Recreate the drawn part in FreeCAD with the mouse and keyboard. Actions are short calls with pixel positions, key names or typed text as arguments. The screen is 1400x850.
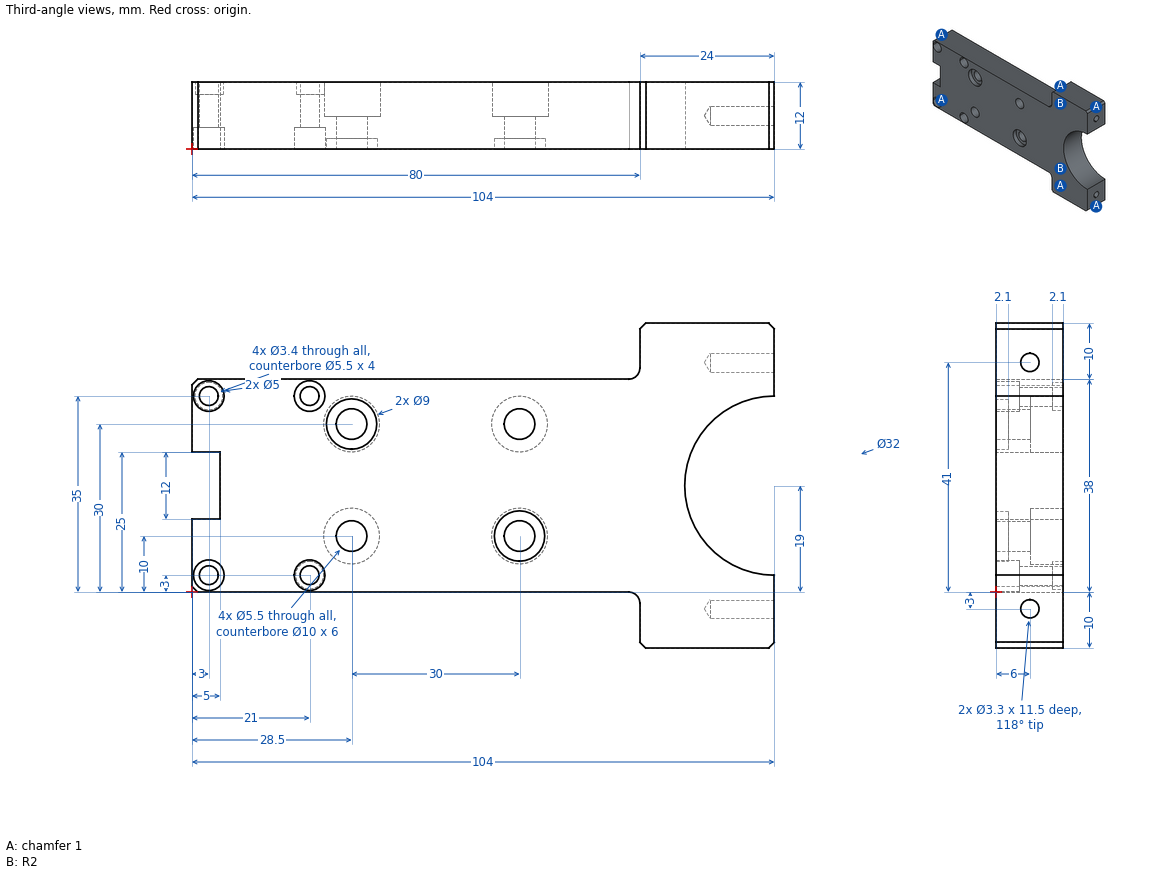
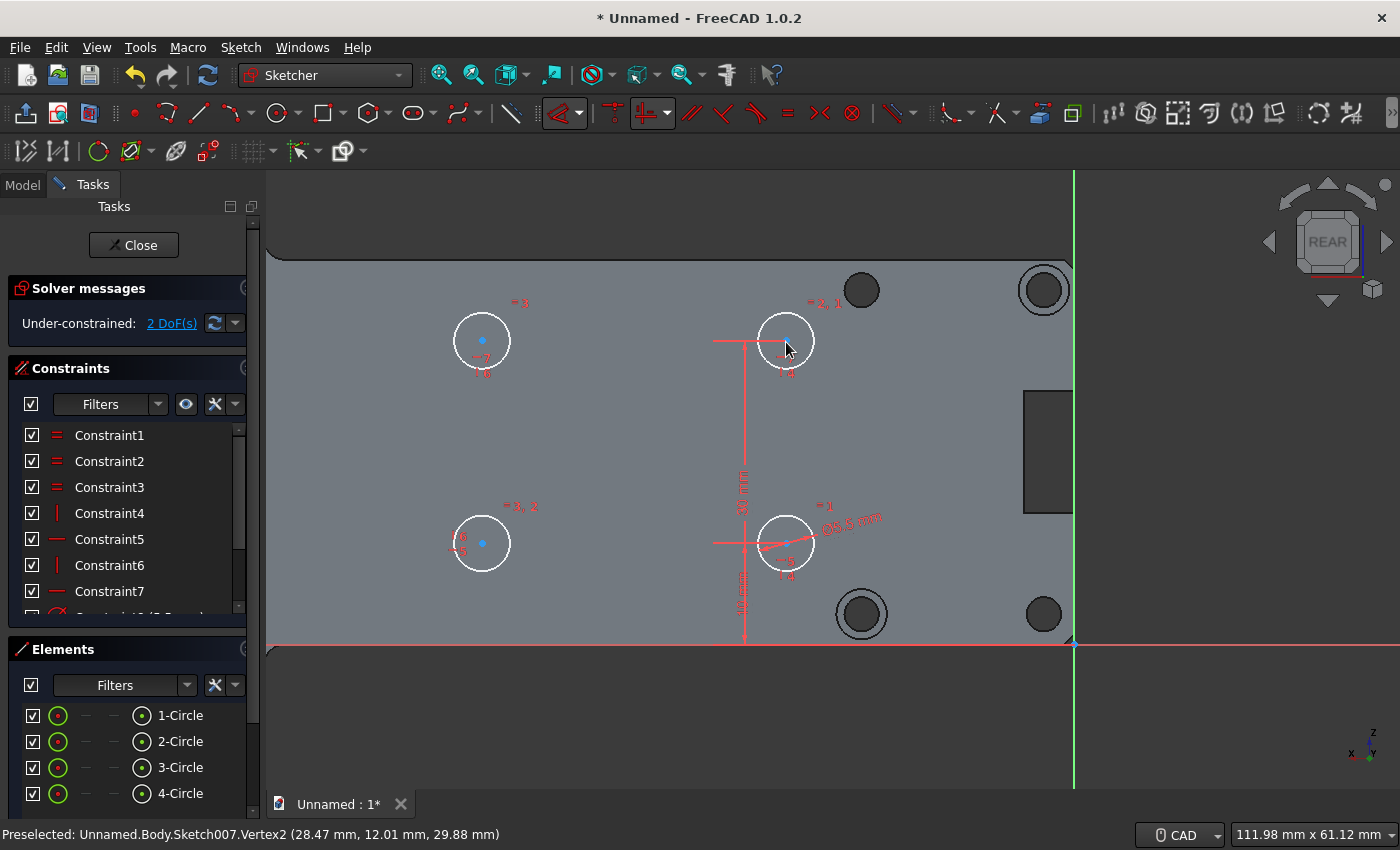
click(786, 543)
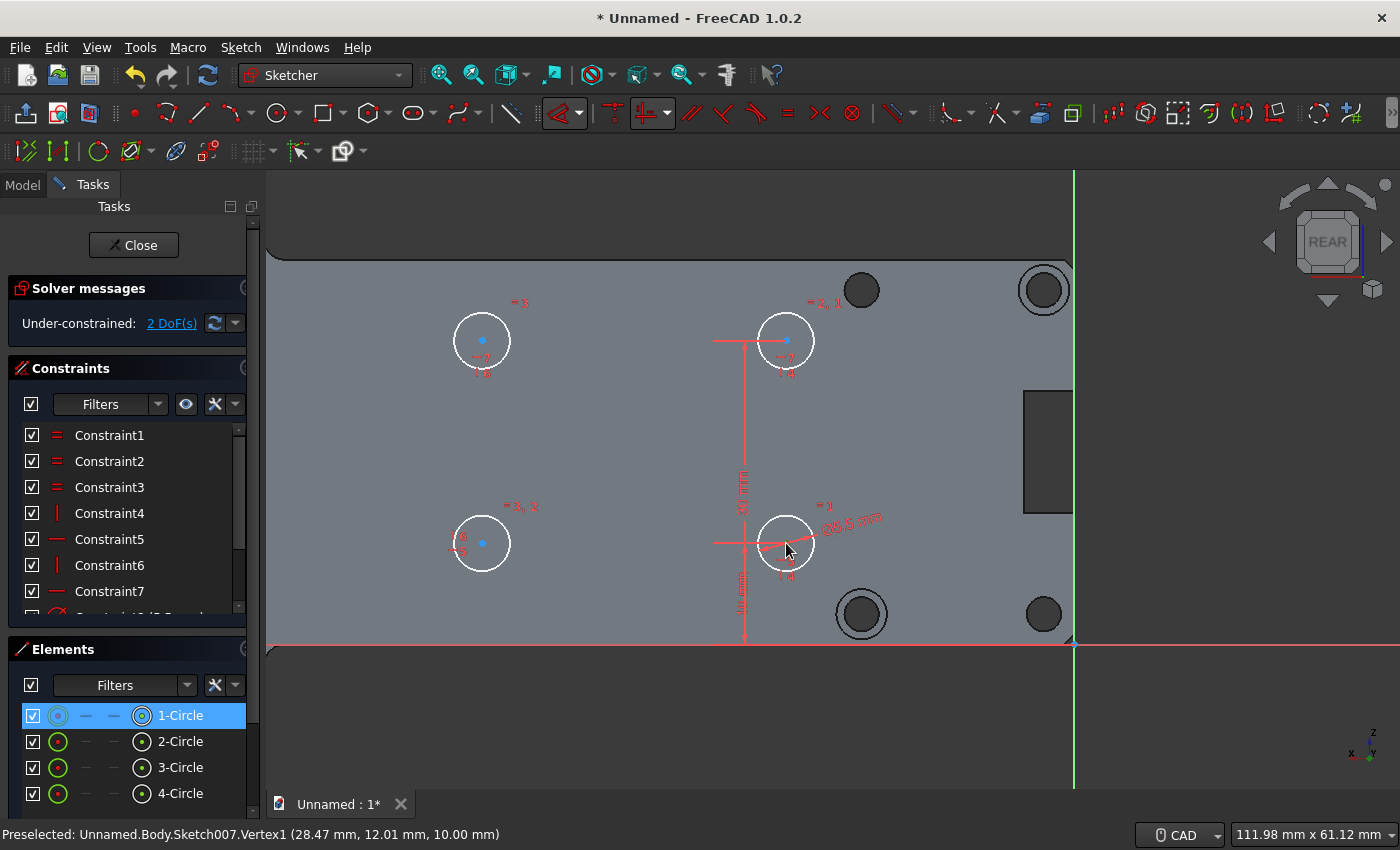
click(482, 543)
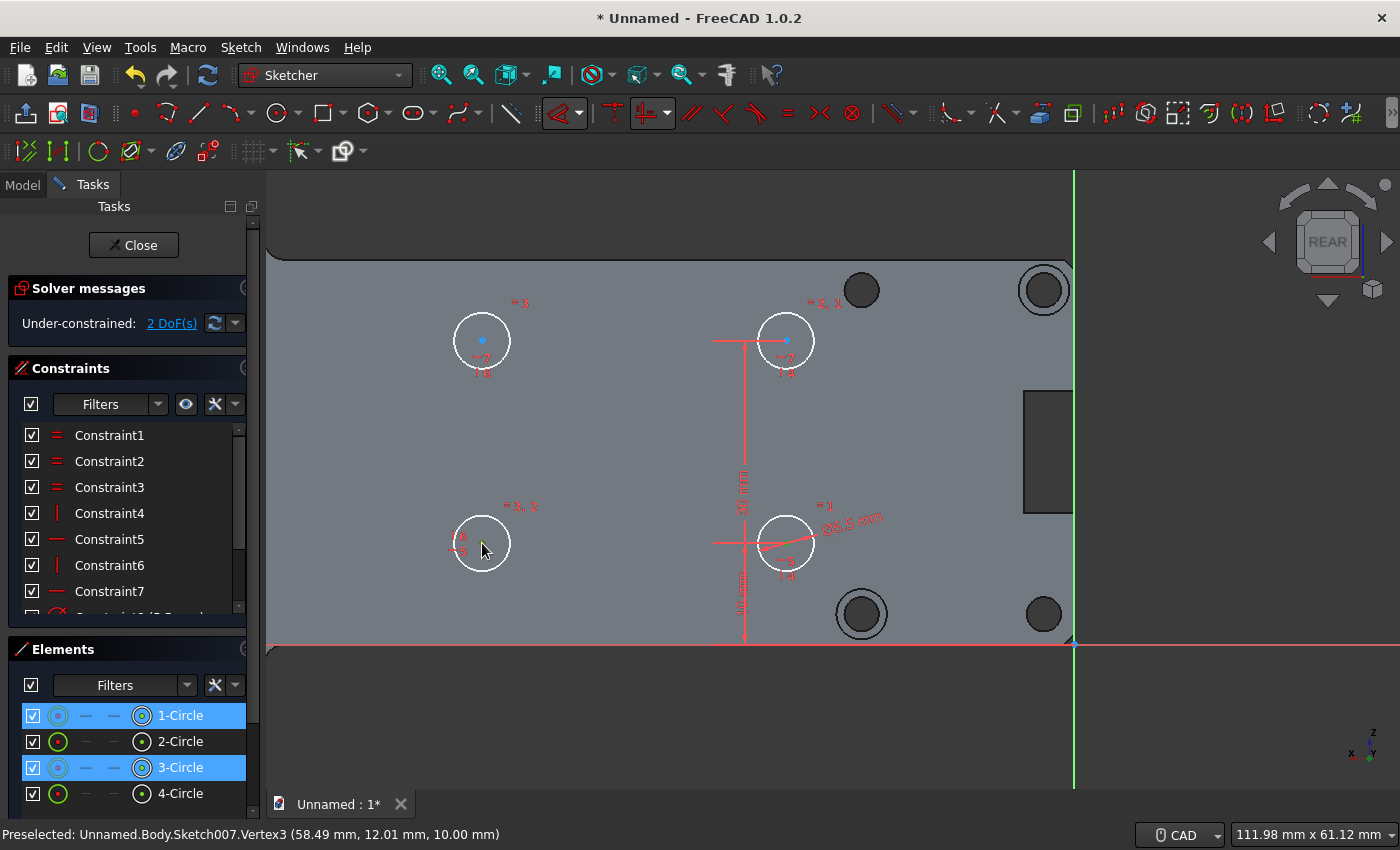
click(582, 114)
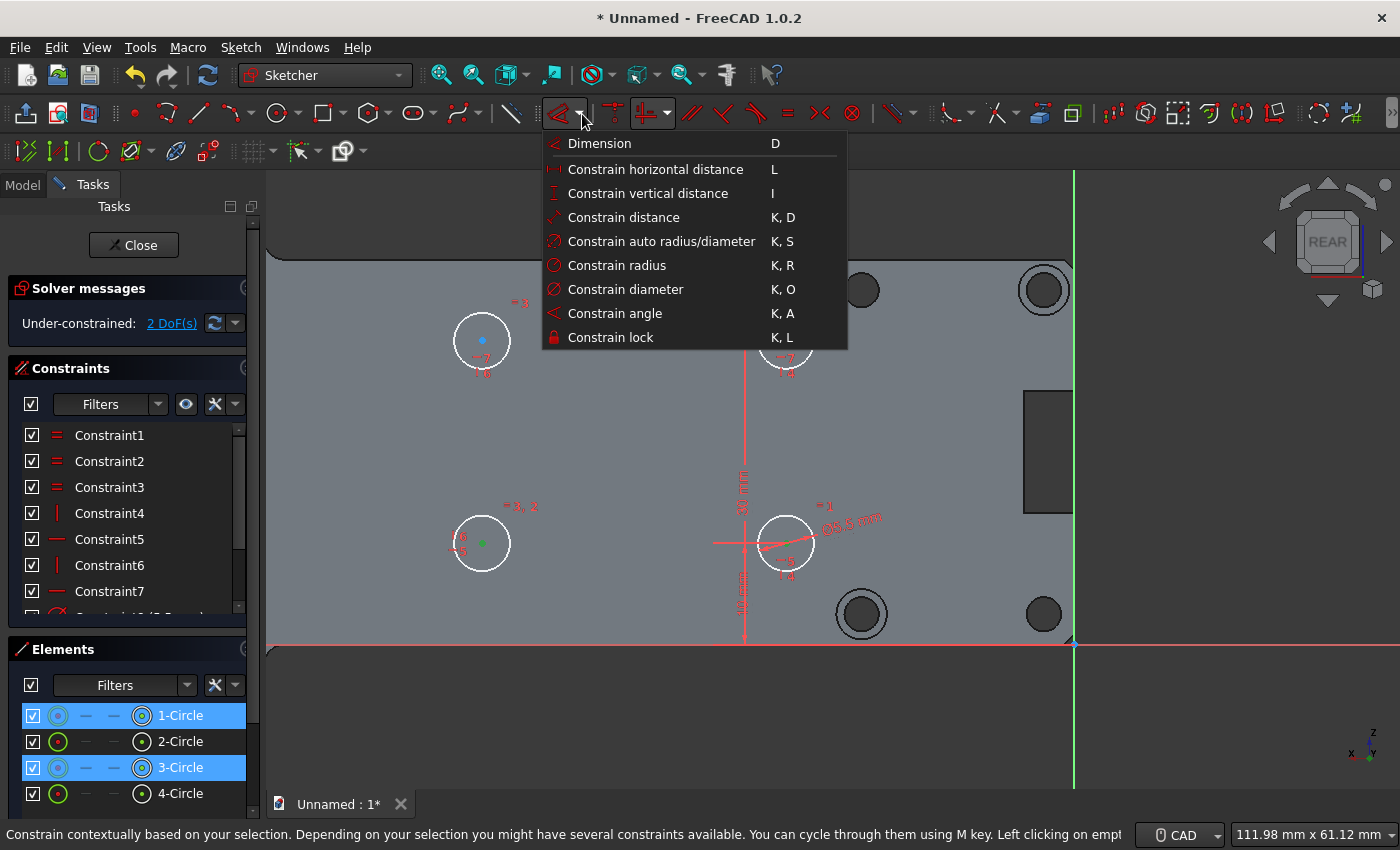
click(695, 169)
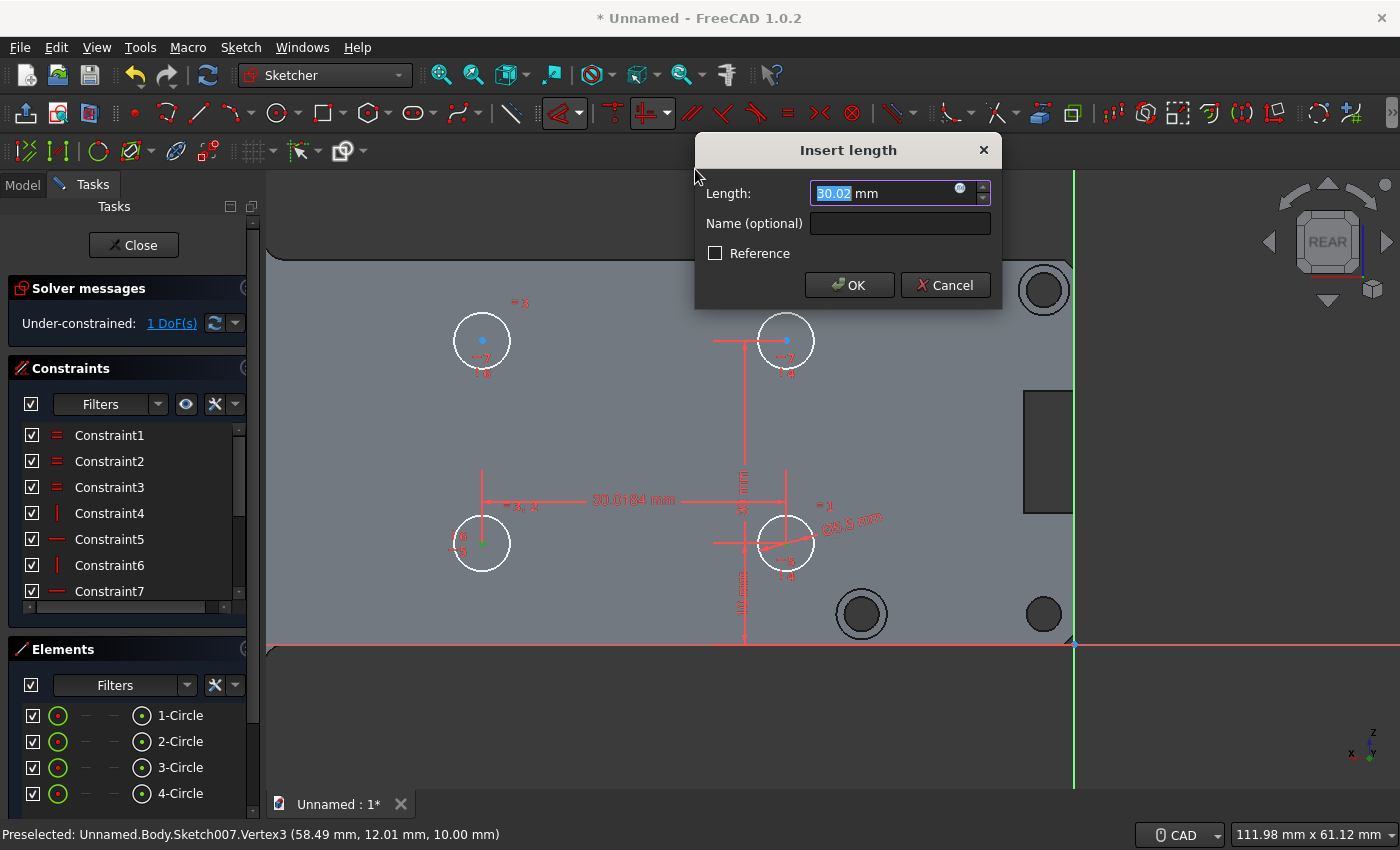
text(30)
key(Return)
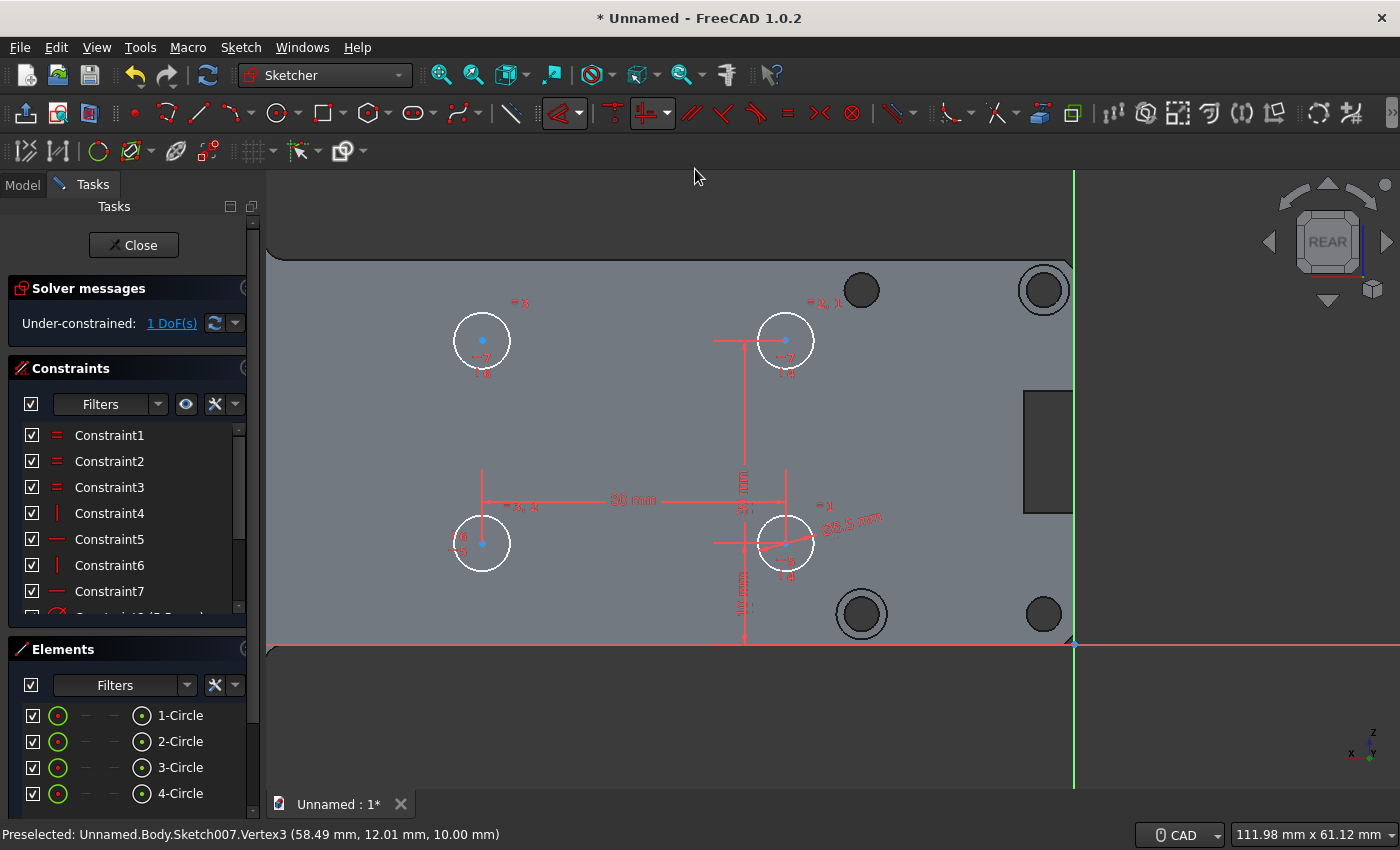
click(786, 543)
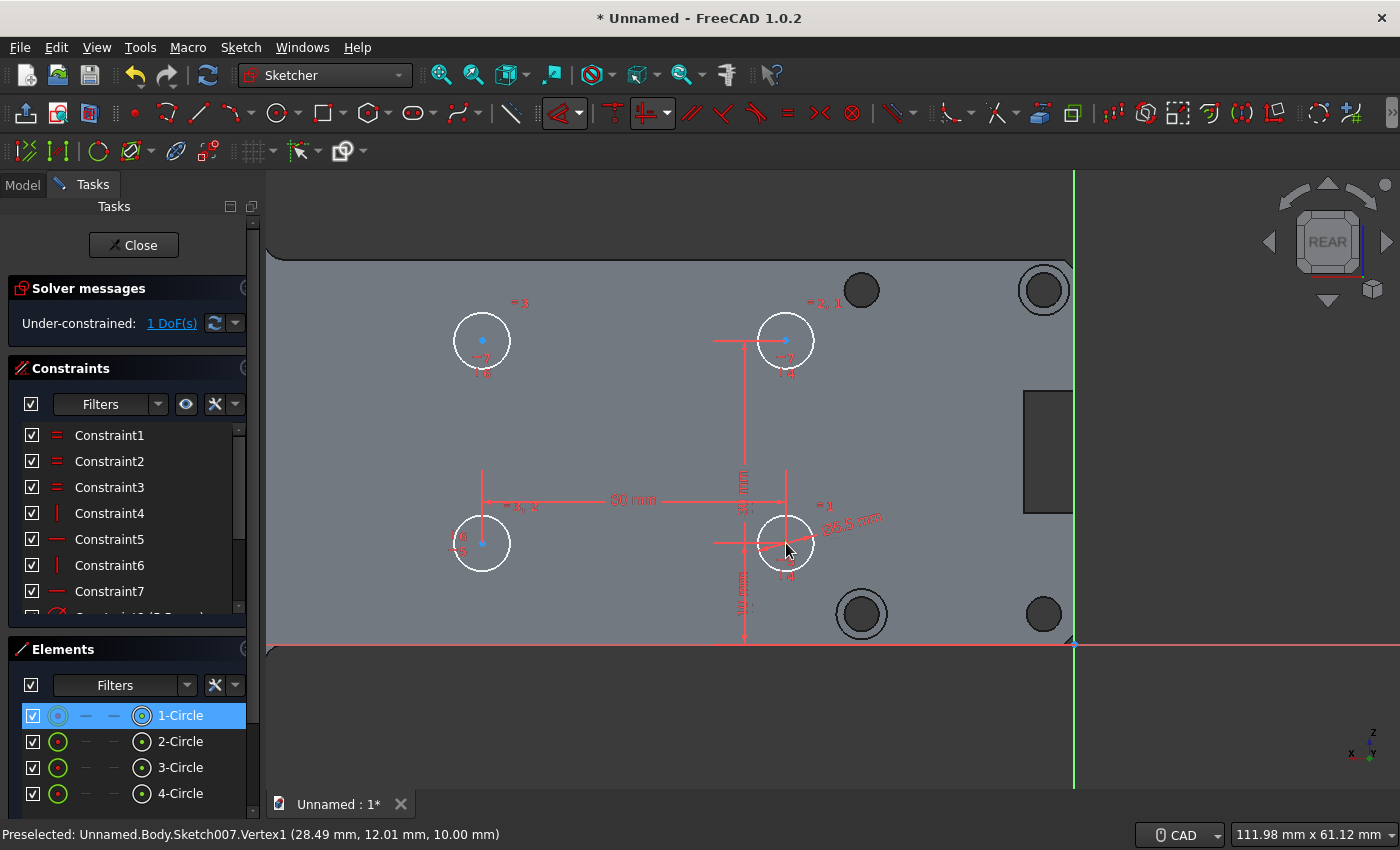
click(582, 114)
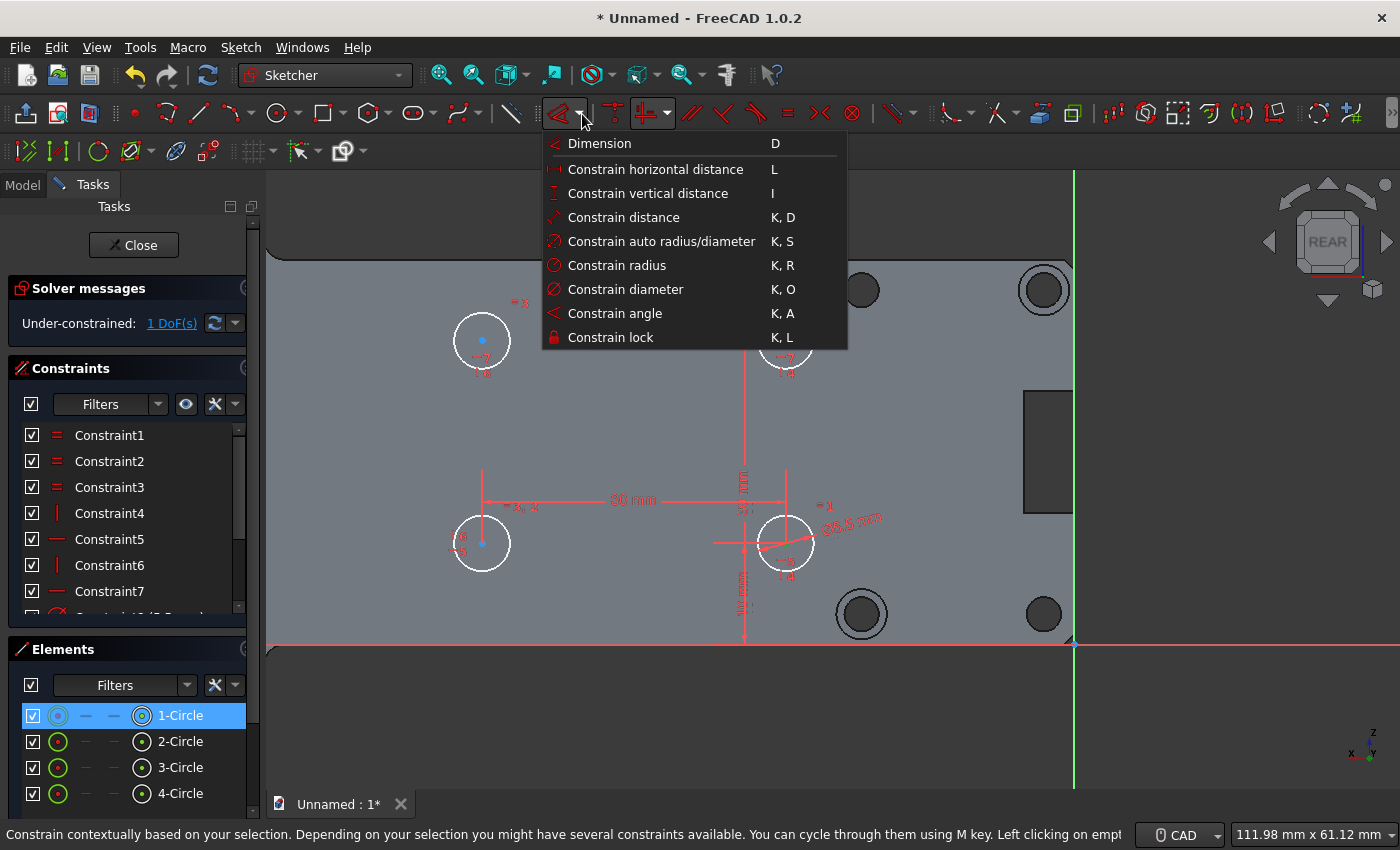
click(695, 169)